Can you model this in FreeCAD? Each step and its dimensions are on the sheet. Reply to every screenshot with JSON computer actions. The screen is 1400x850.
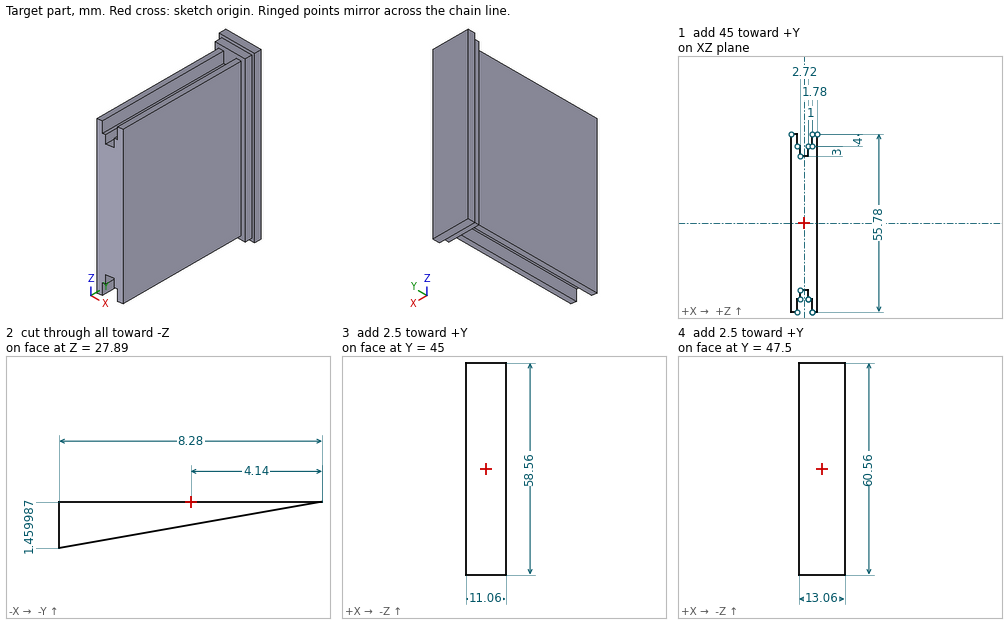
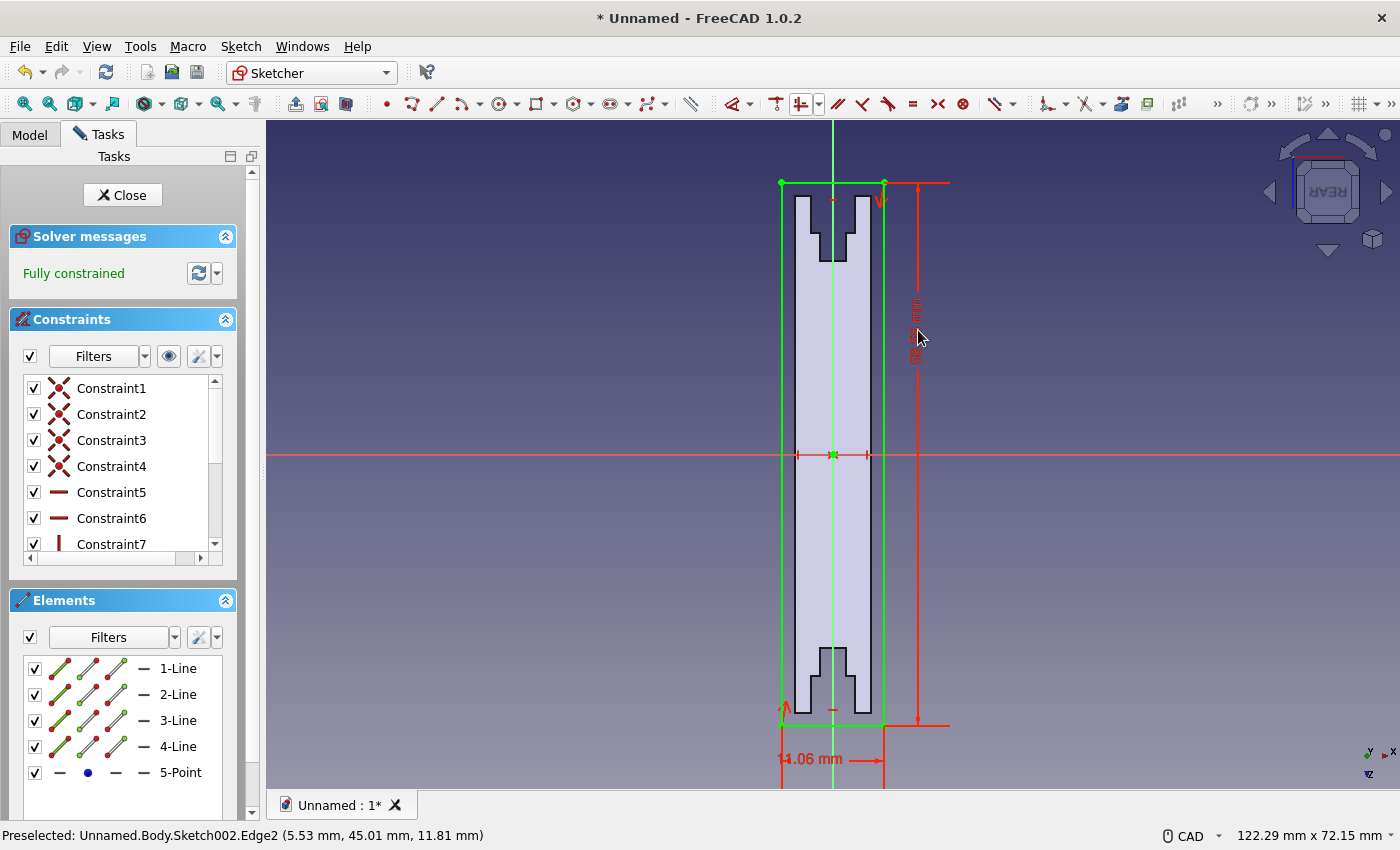
{"action": "left_click", "coordinate": [123, 195]}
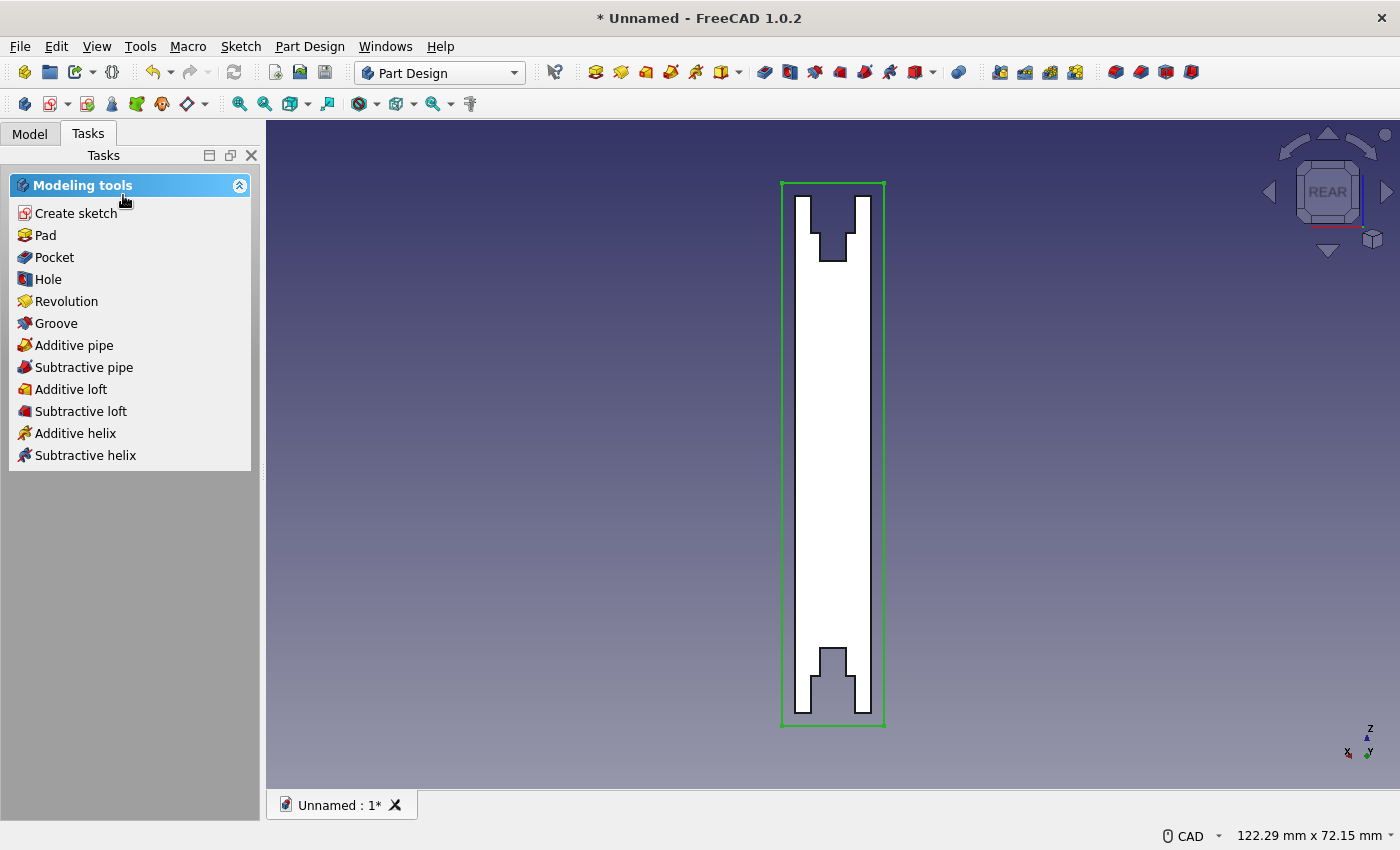
{"action": "left_click", "coordinate": [596, 72]}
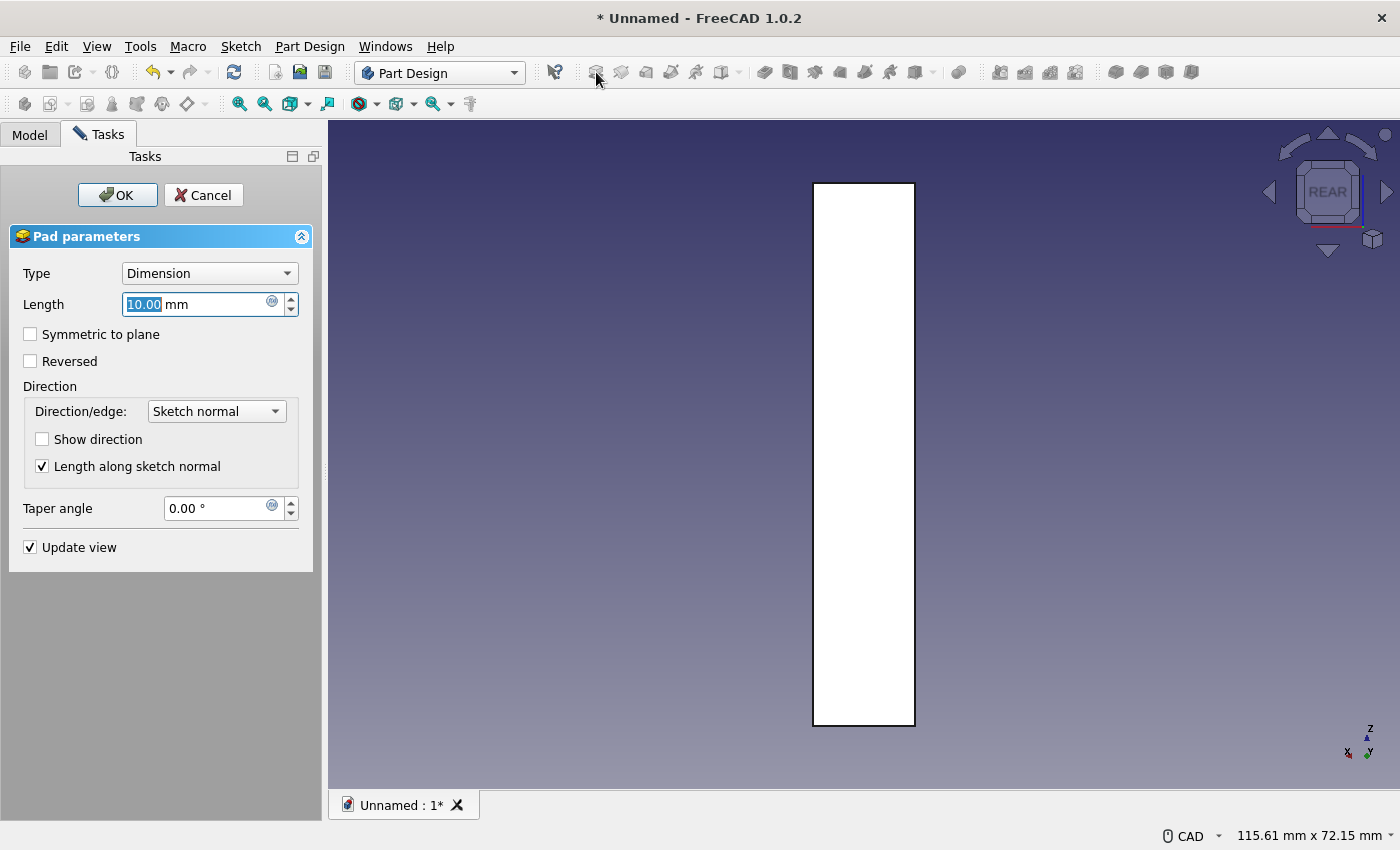
{"action": "type", "text": "2.5"}
{"action": "key", "text": "Tab"}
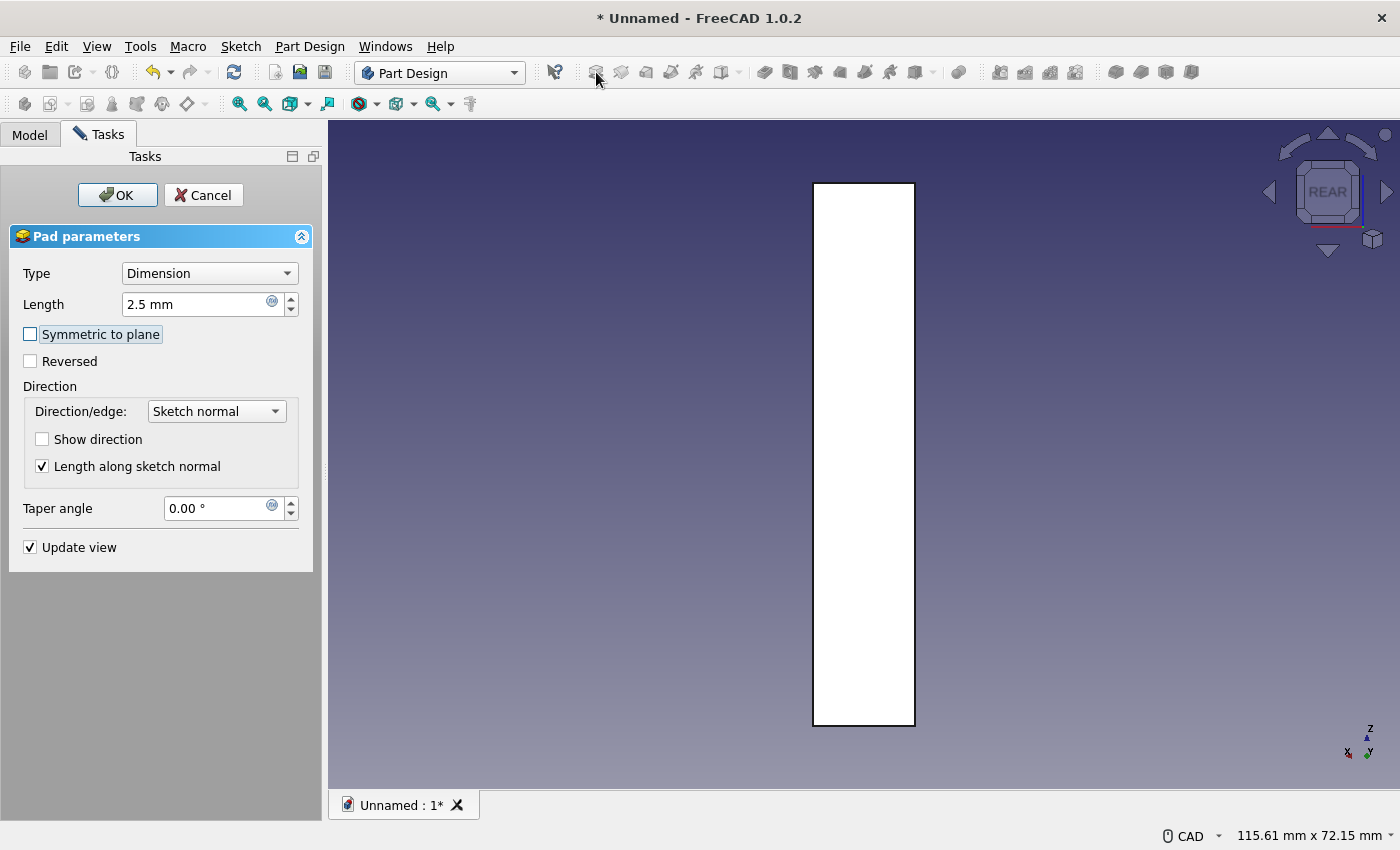
{"action": "left_click", "coordinate": [118, 195]}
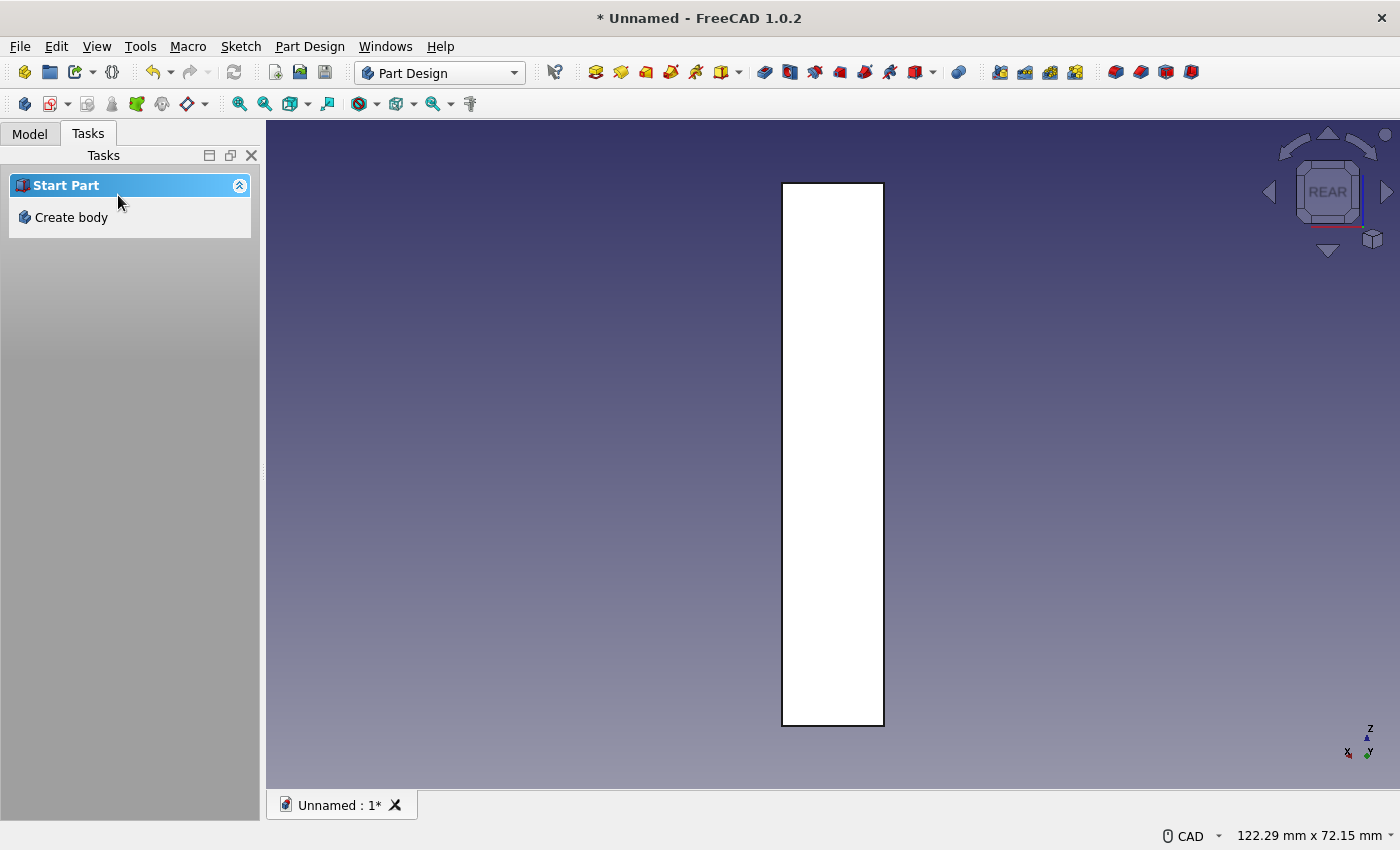
{"action": "left_click", "coordinate": [833, 609]}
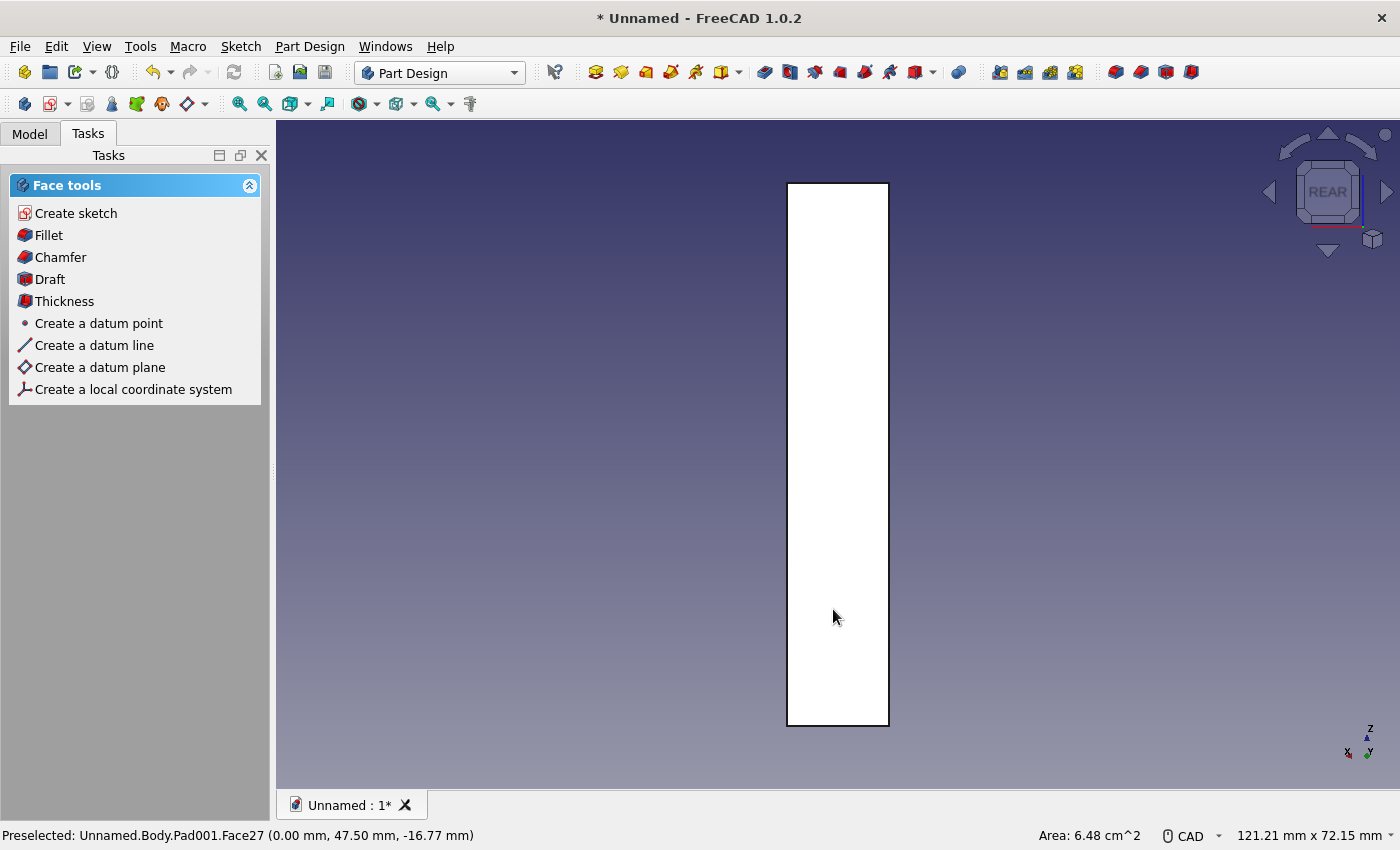
{"action": "left_click", "coordinate": [50, 104]}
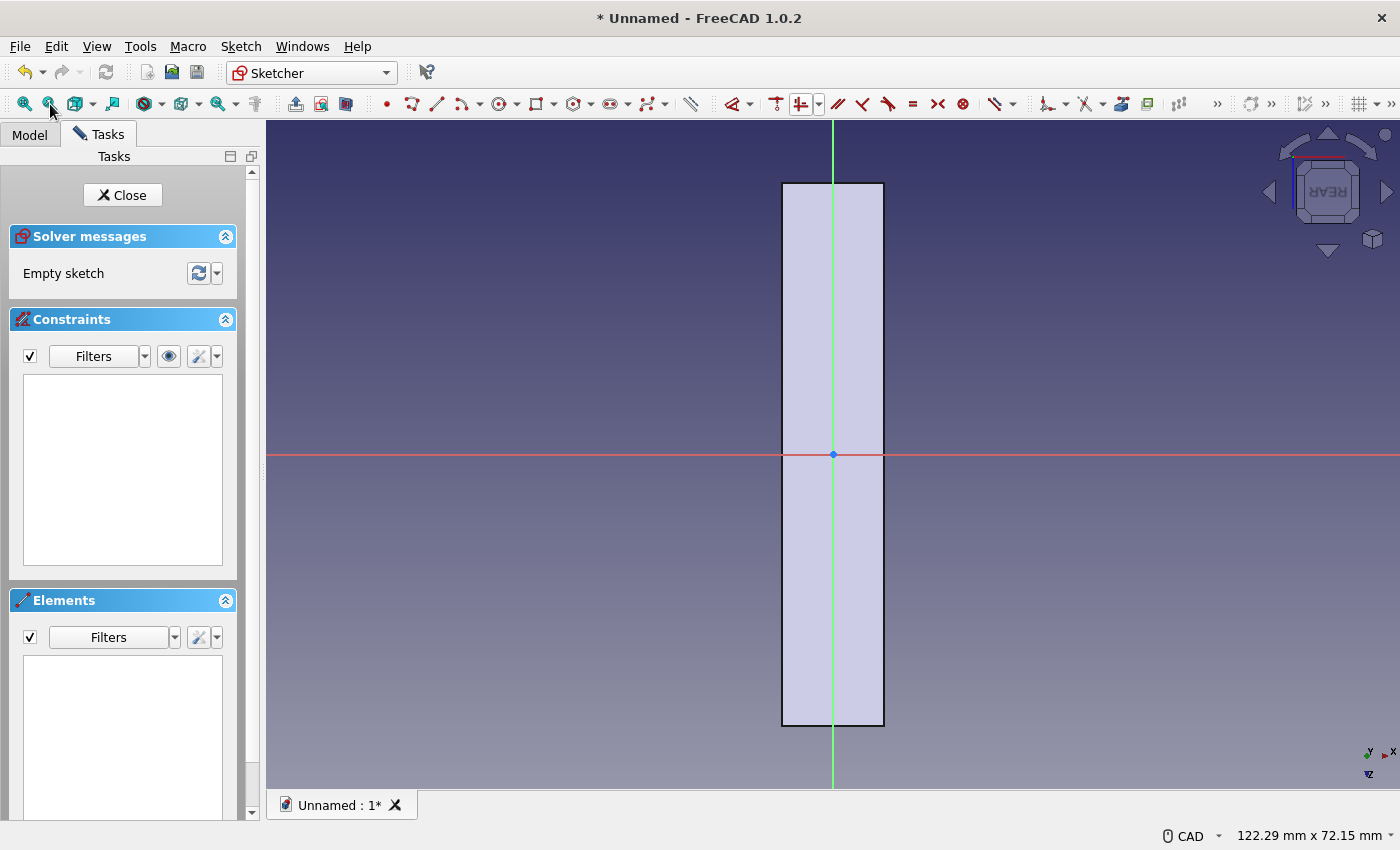
{"action": "left_click", "coordinate": [554, 104]}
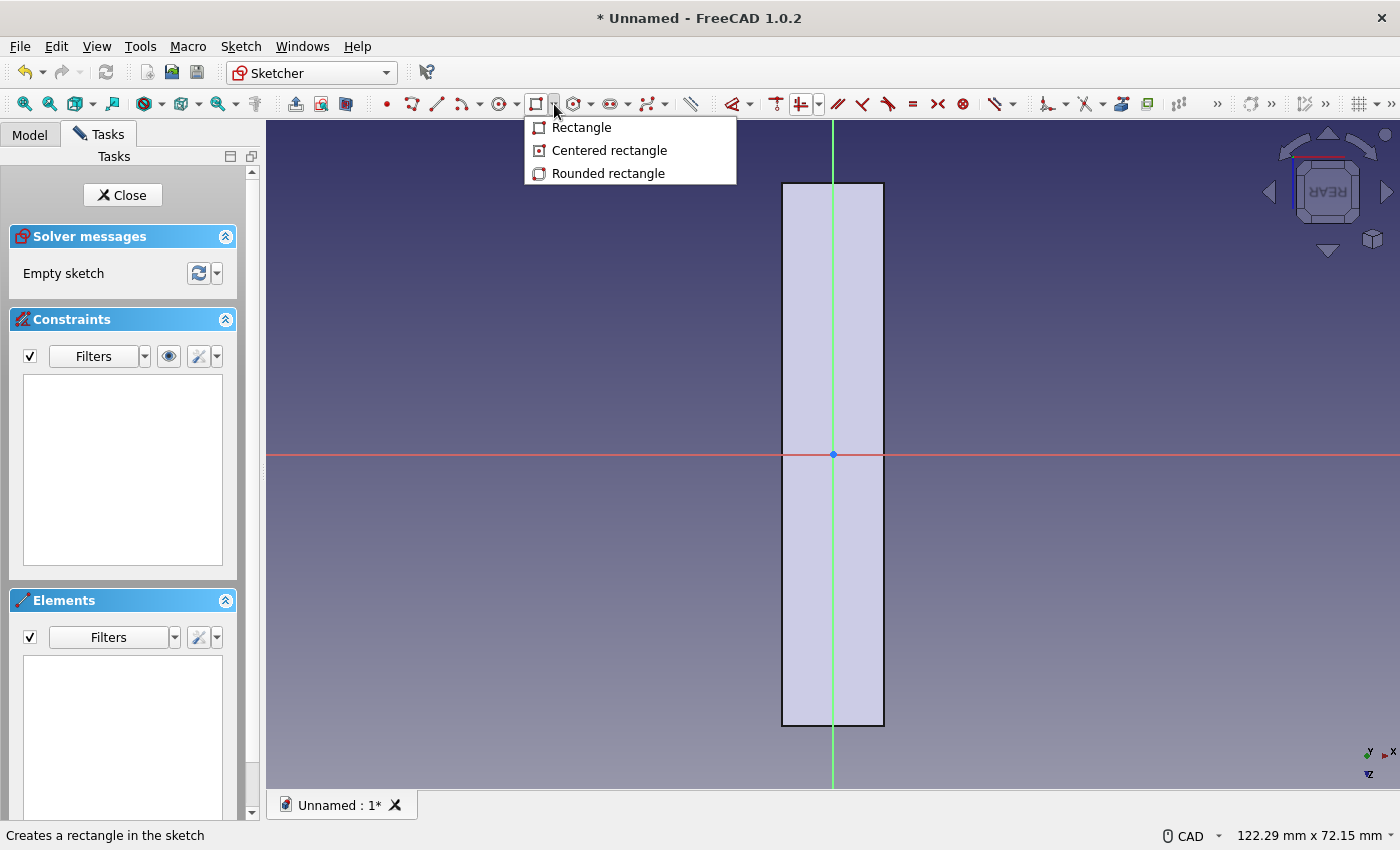
{"action": "left_click", "coordinate": [630, 150]}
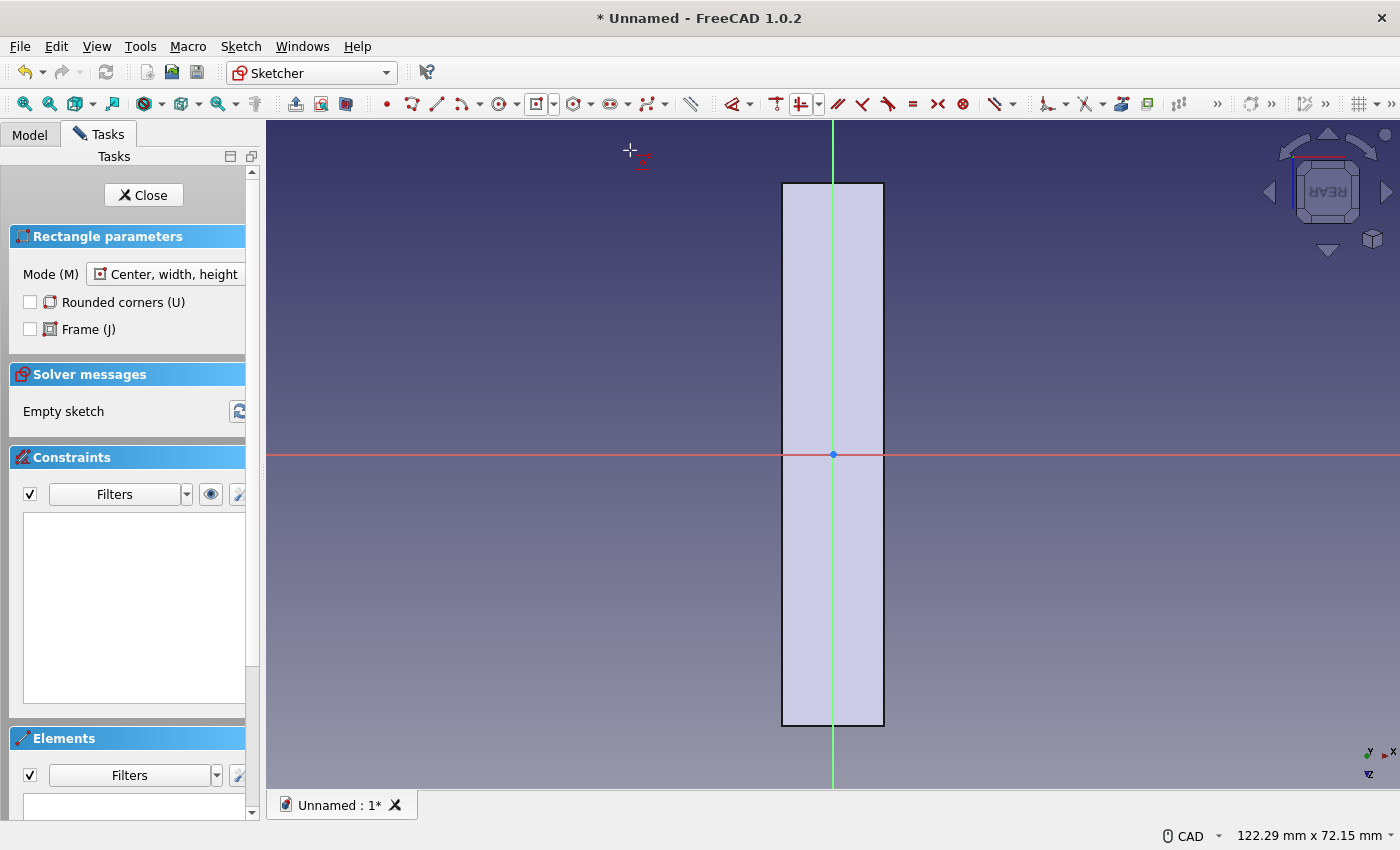
{"action": "left_click", "coordinate": [833, 454]}
{"action": "left_click", "coordinate": [894, 174]}
{"action": "key", "text": "Escape"}